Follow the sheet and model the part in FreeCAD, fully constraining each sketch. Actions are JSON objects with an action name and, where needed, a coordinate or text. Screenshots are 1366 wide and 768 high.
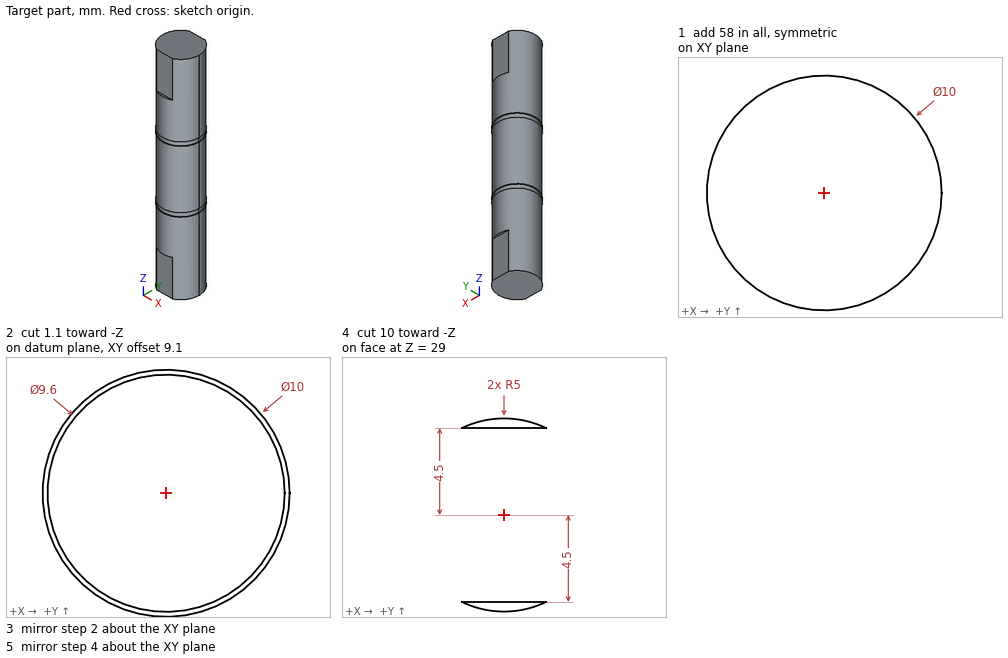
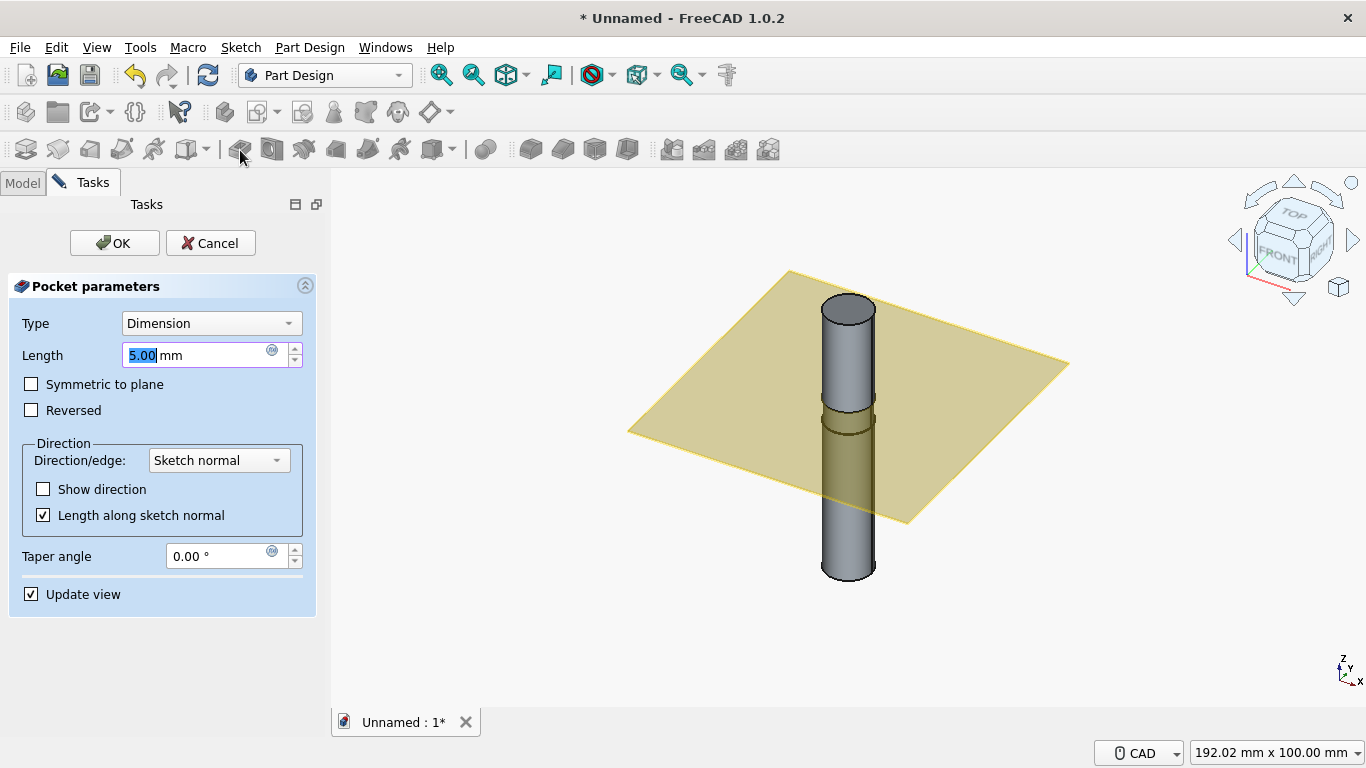
{"action": "type", "text": "1.1"}
{"action": "key", "text": "Tab"}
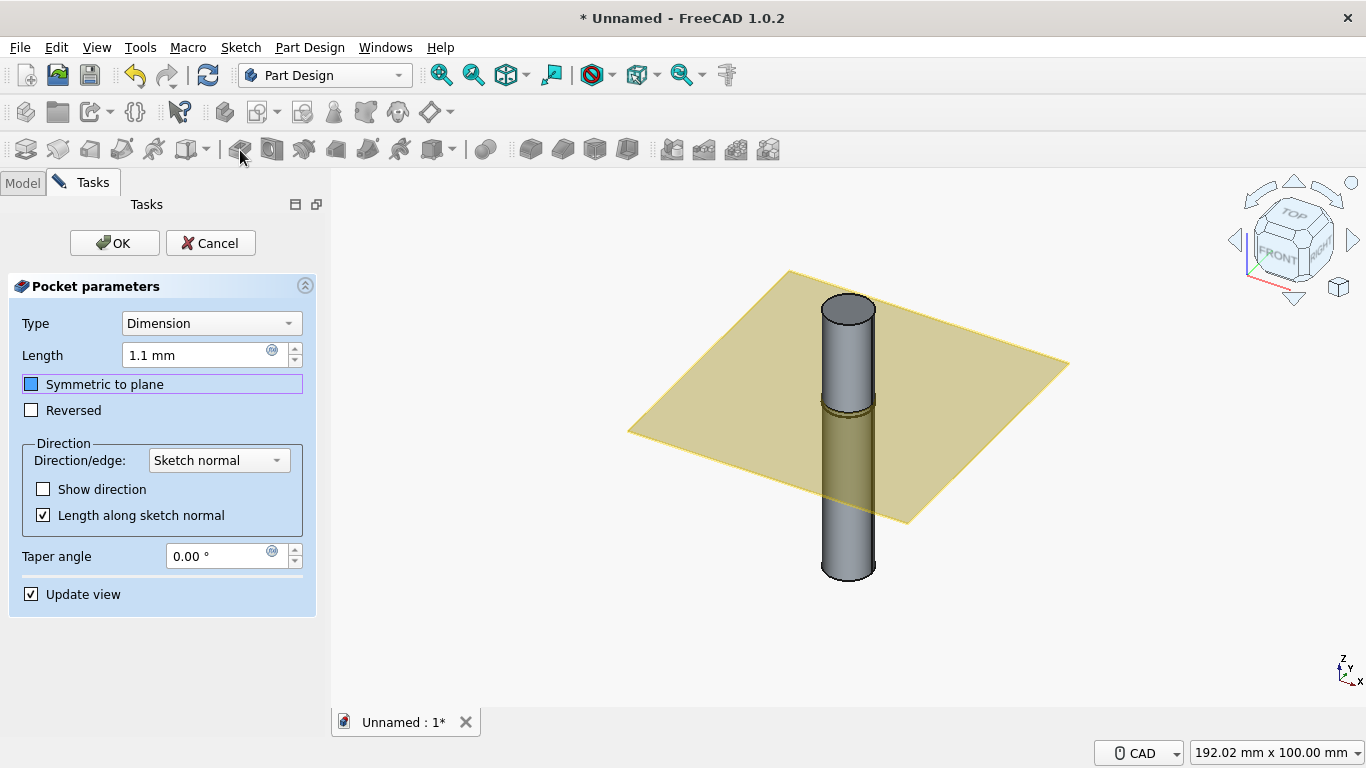
{"action": "left_click", "coordinate": [115, 243]}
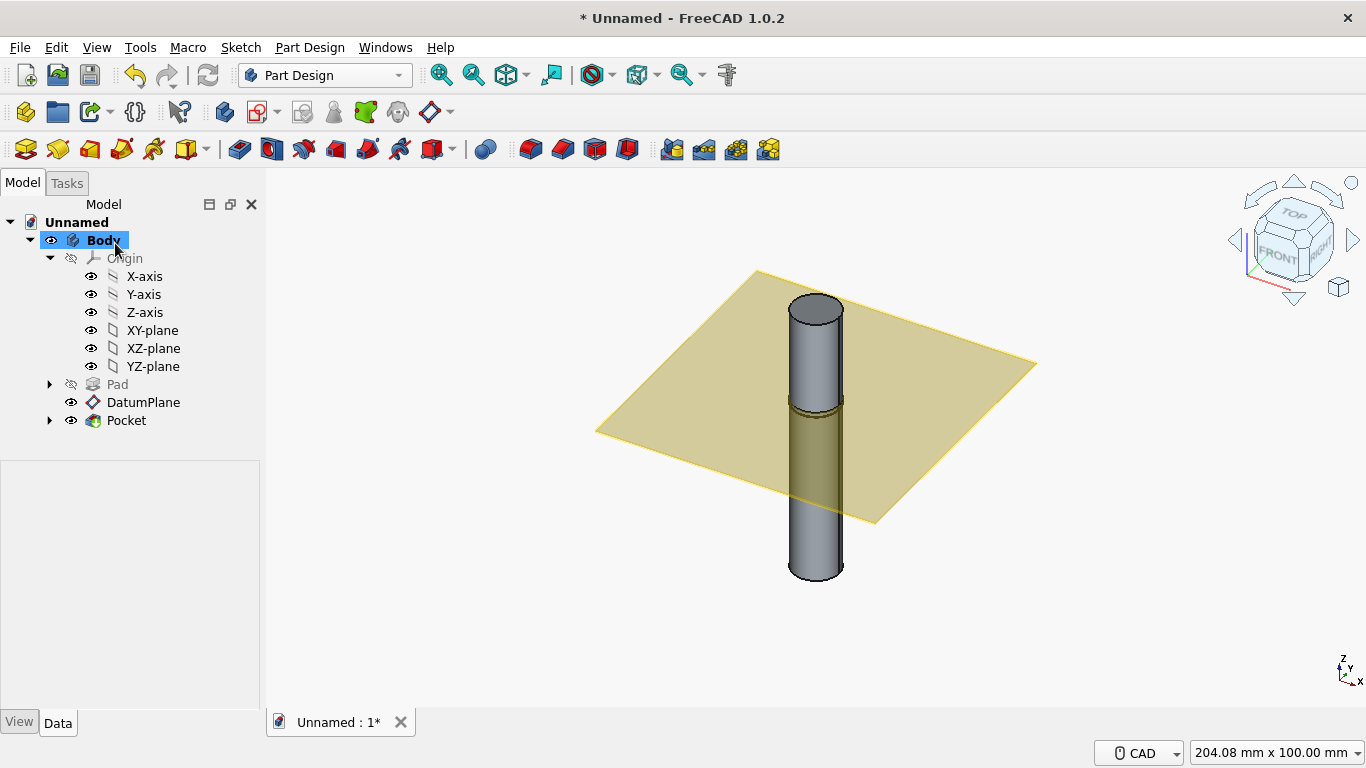
{"action": "left_click", "coordinate": [116, 402]}
{"action": "key", "text": "space"}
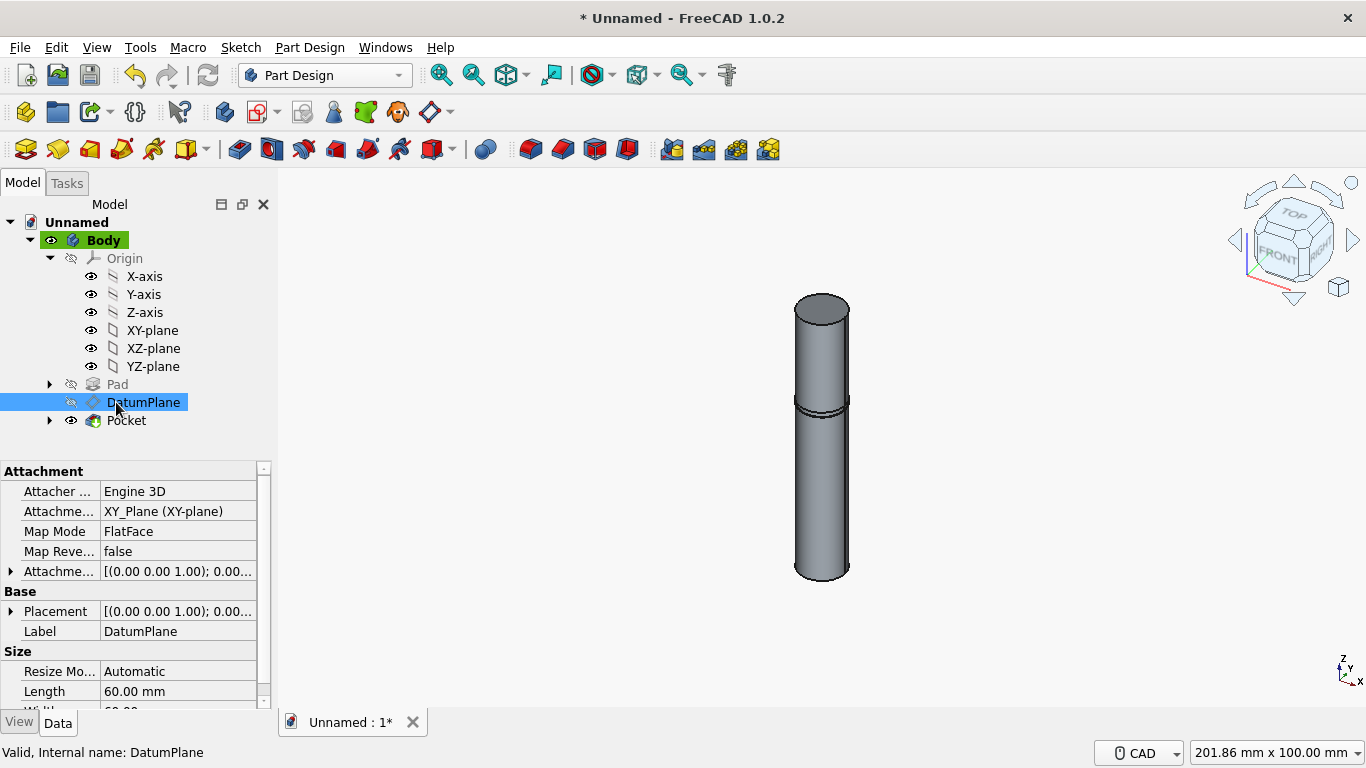
{"action": "left_click", "coordinate": [116, 420]}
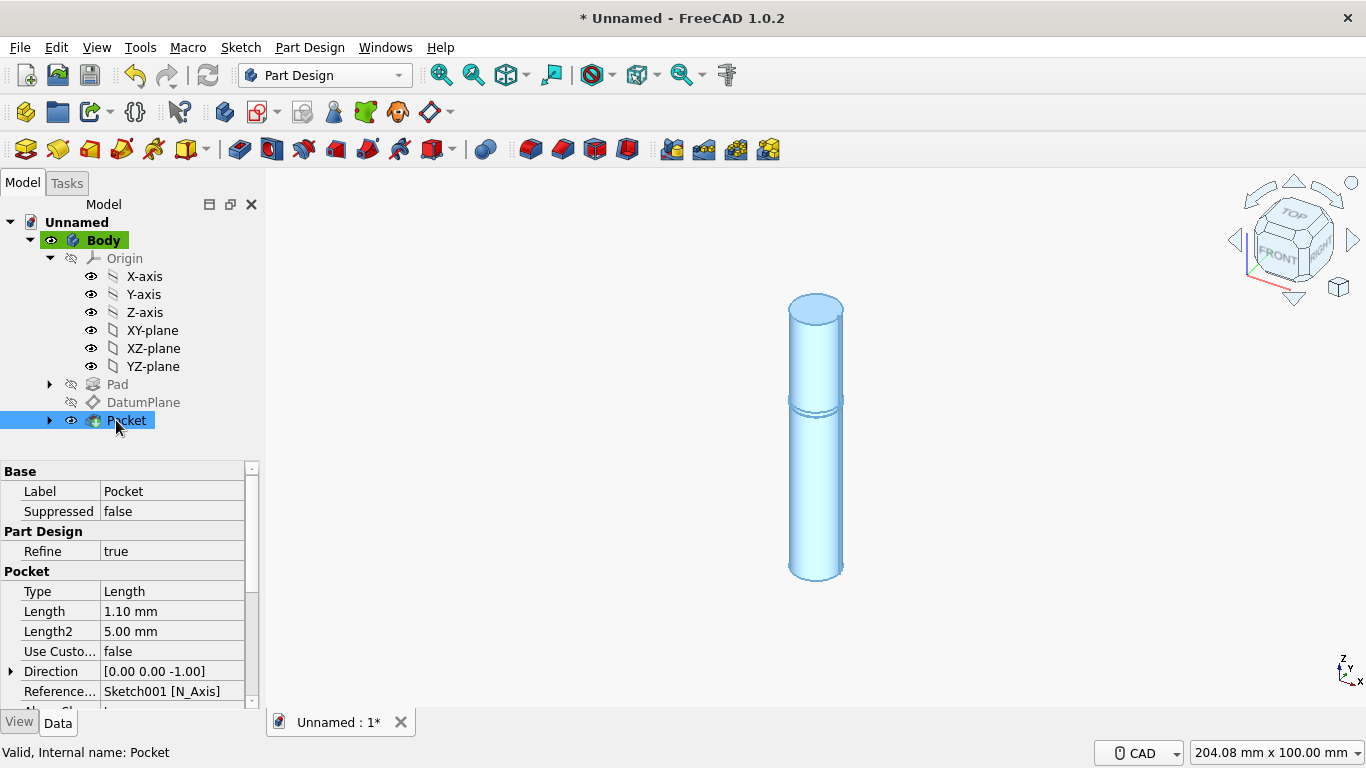
{"action": "left_click", "coordinate": [672, 150]}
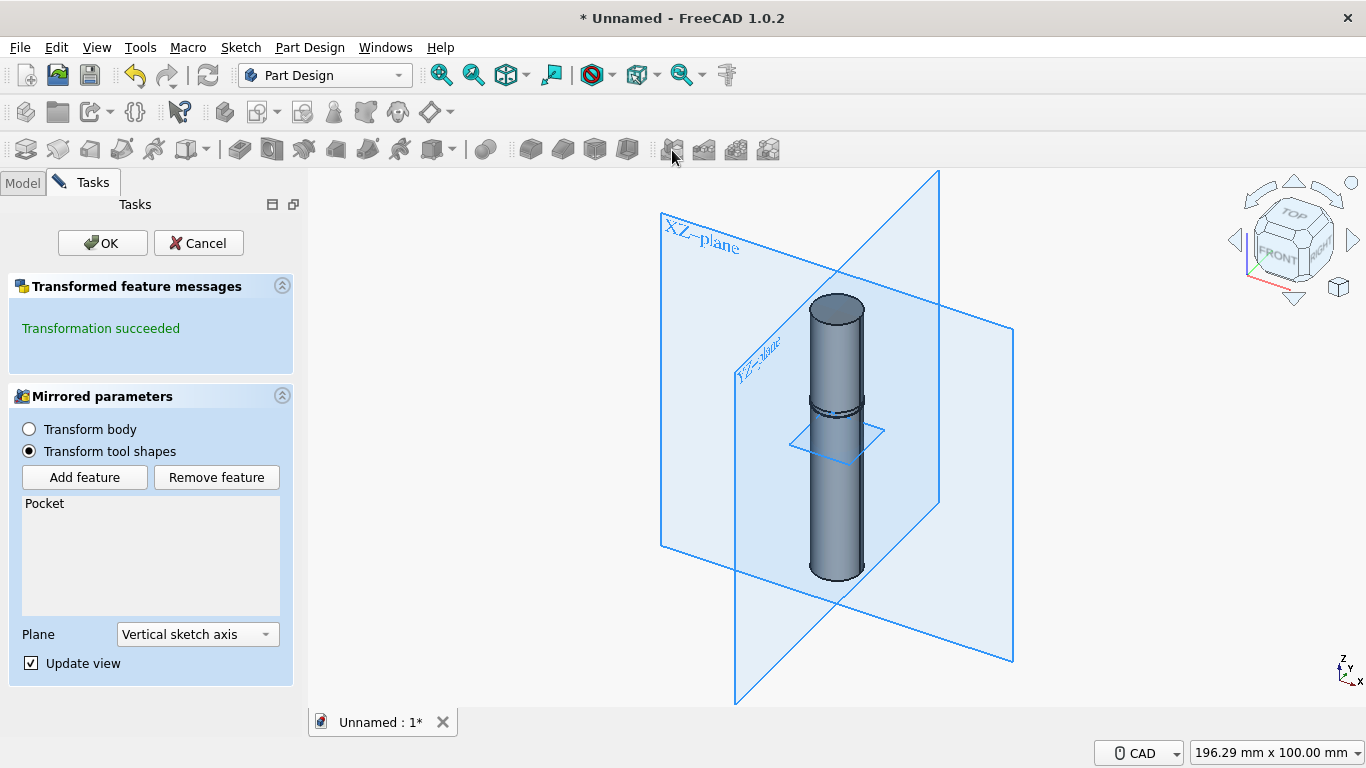
{"action": "left_click", "coordinate": [198, 634]}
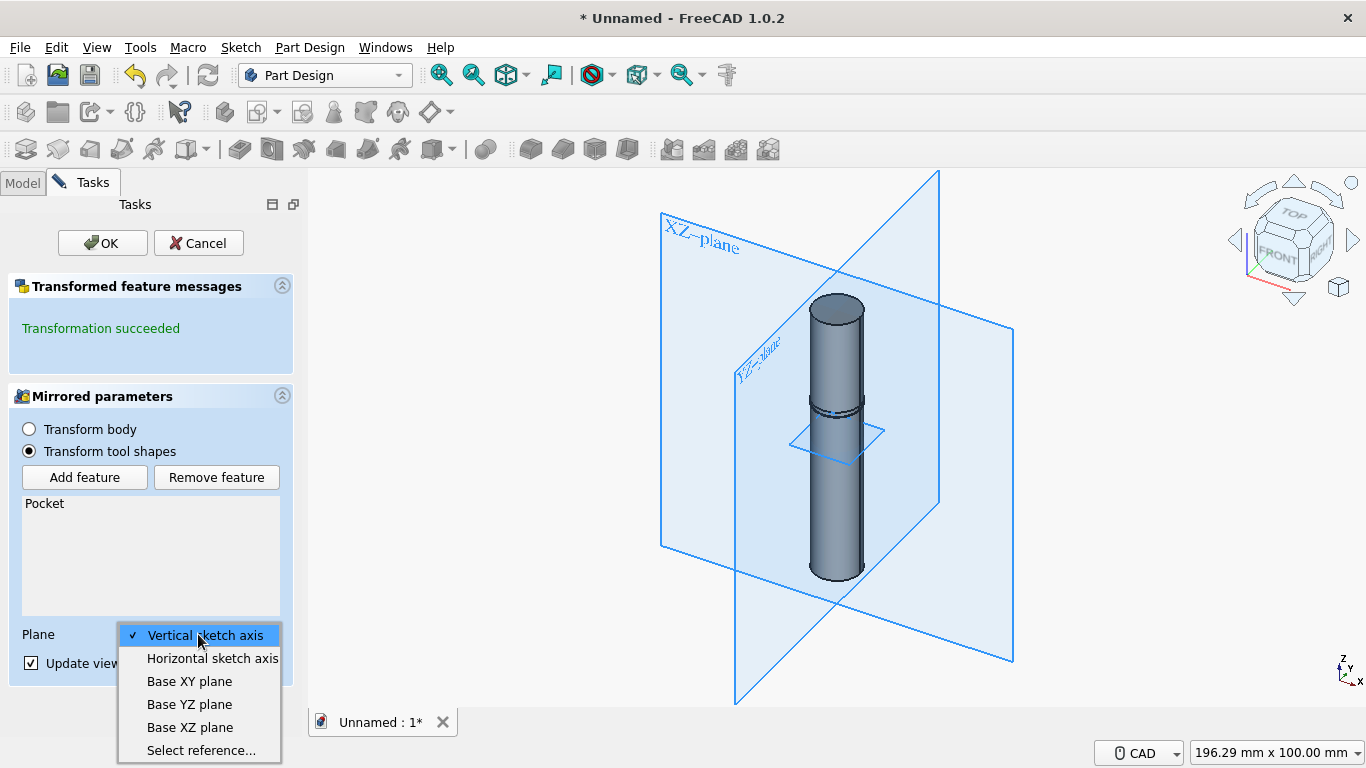
{"action": "left_click", "coordinate": [198, 682]}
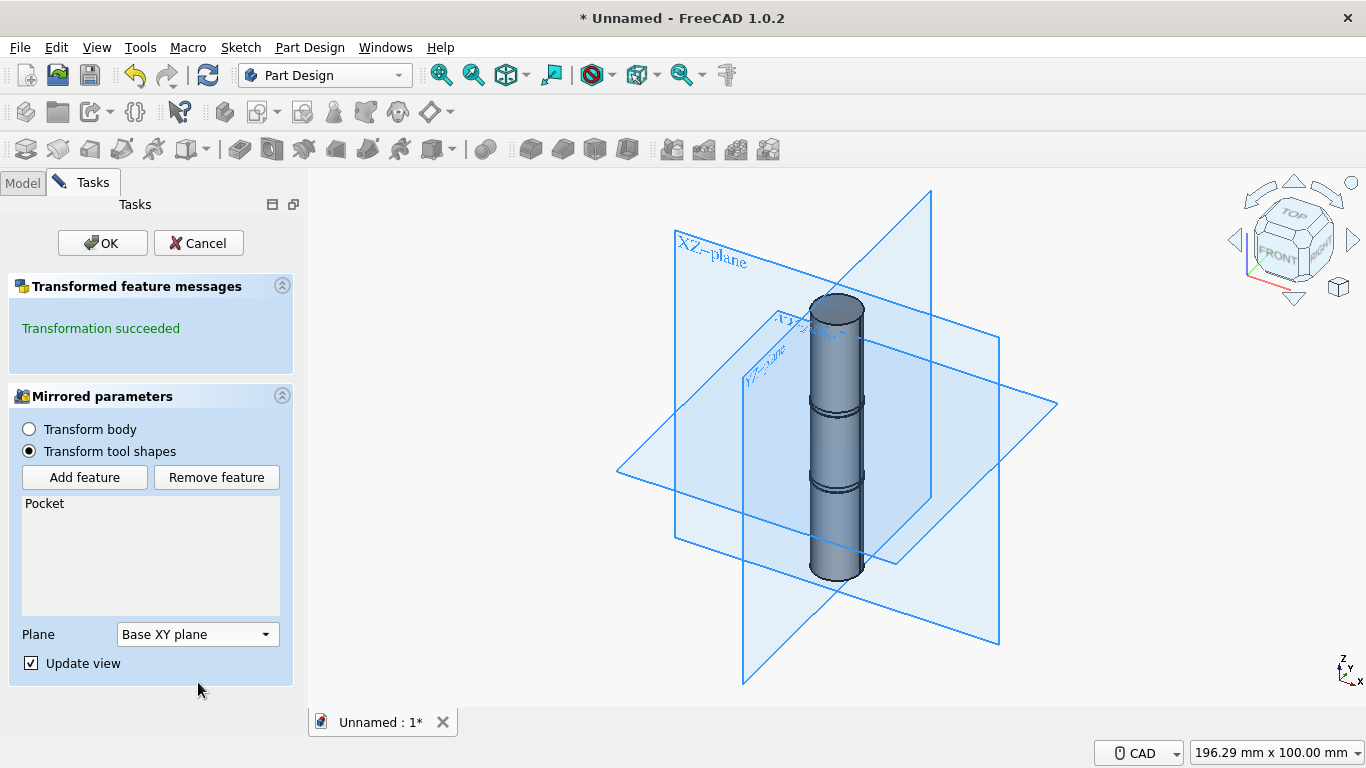
{"action": "left_click", "coordinate": [103, 243]}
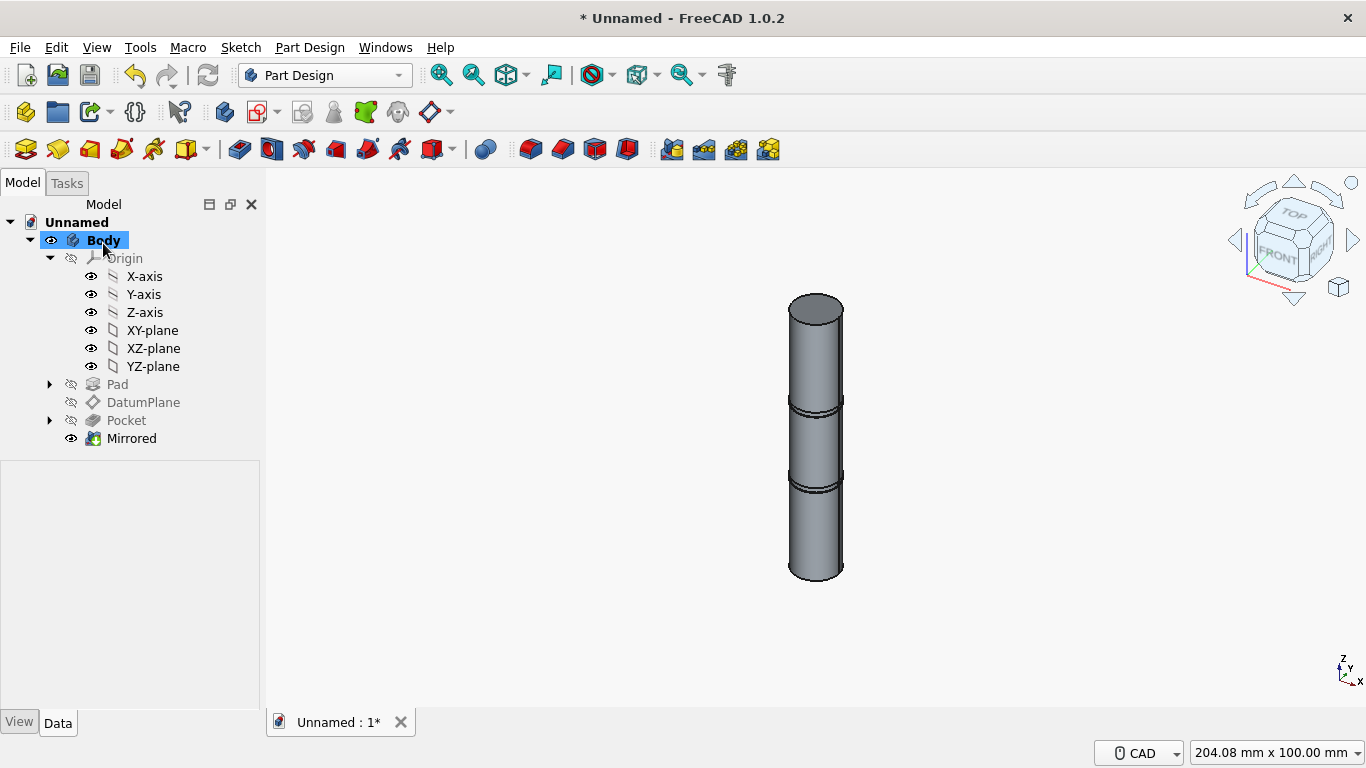
{"action": "left_click", "coordinate": [816, 308]}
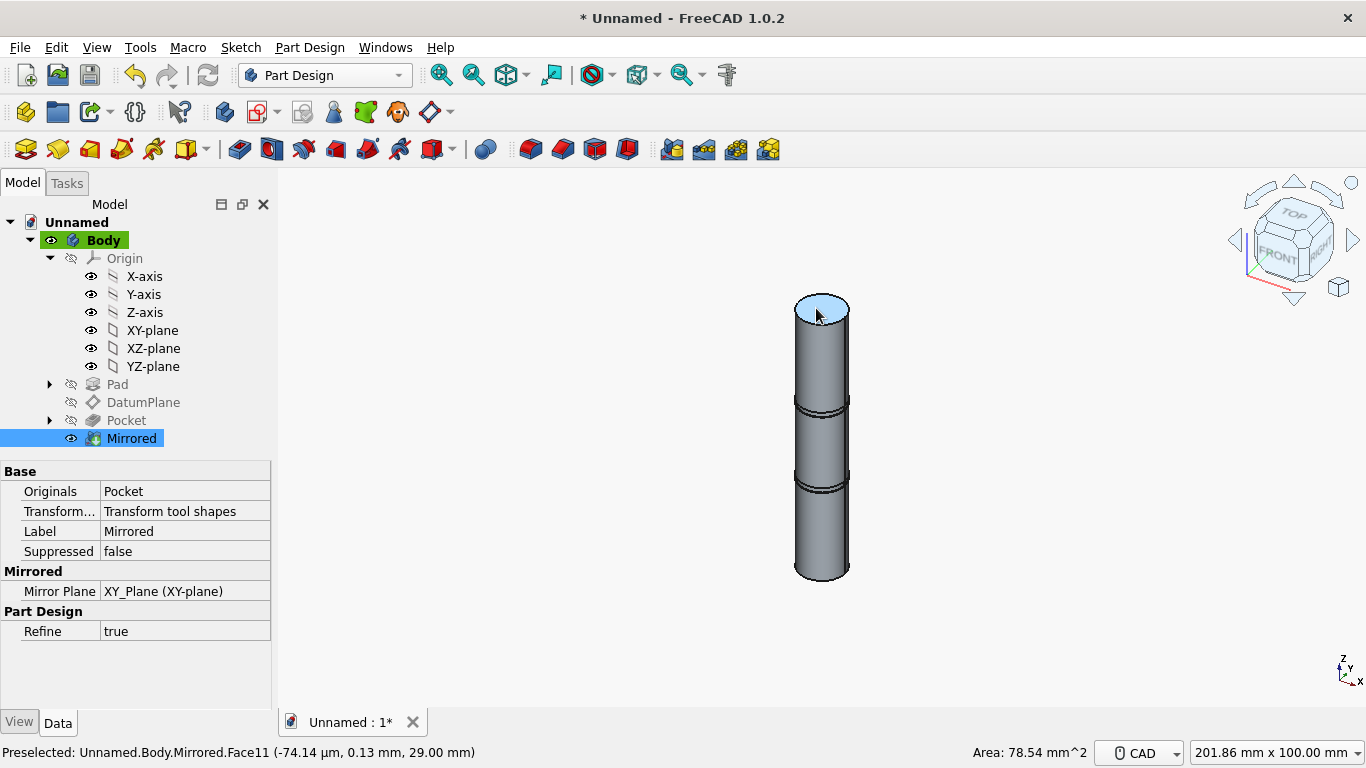
{"action": "left_click", "coordinate": [258, 112]}